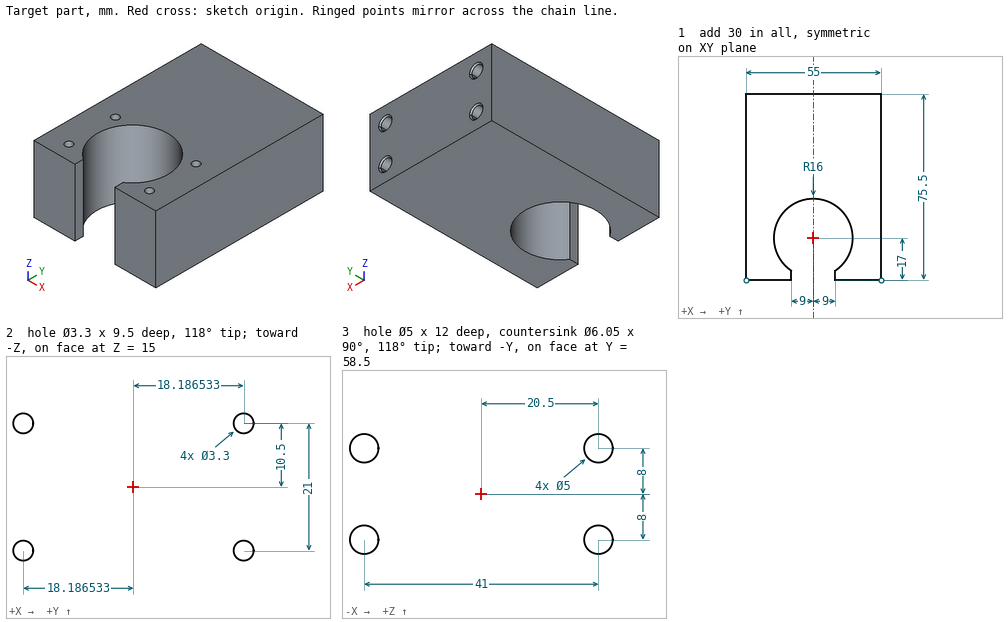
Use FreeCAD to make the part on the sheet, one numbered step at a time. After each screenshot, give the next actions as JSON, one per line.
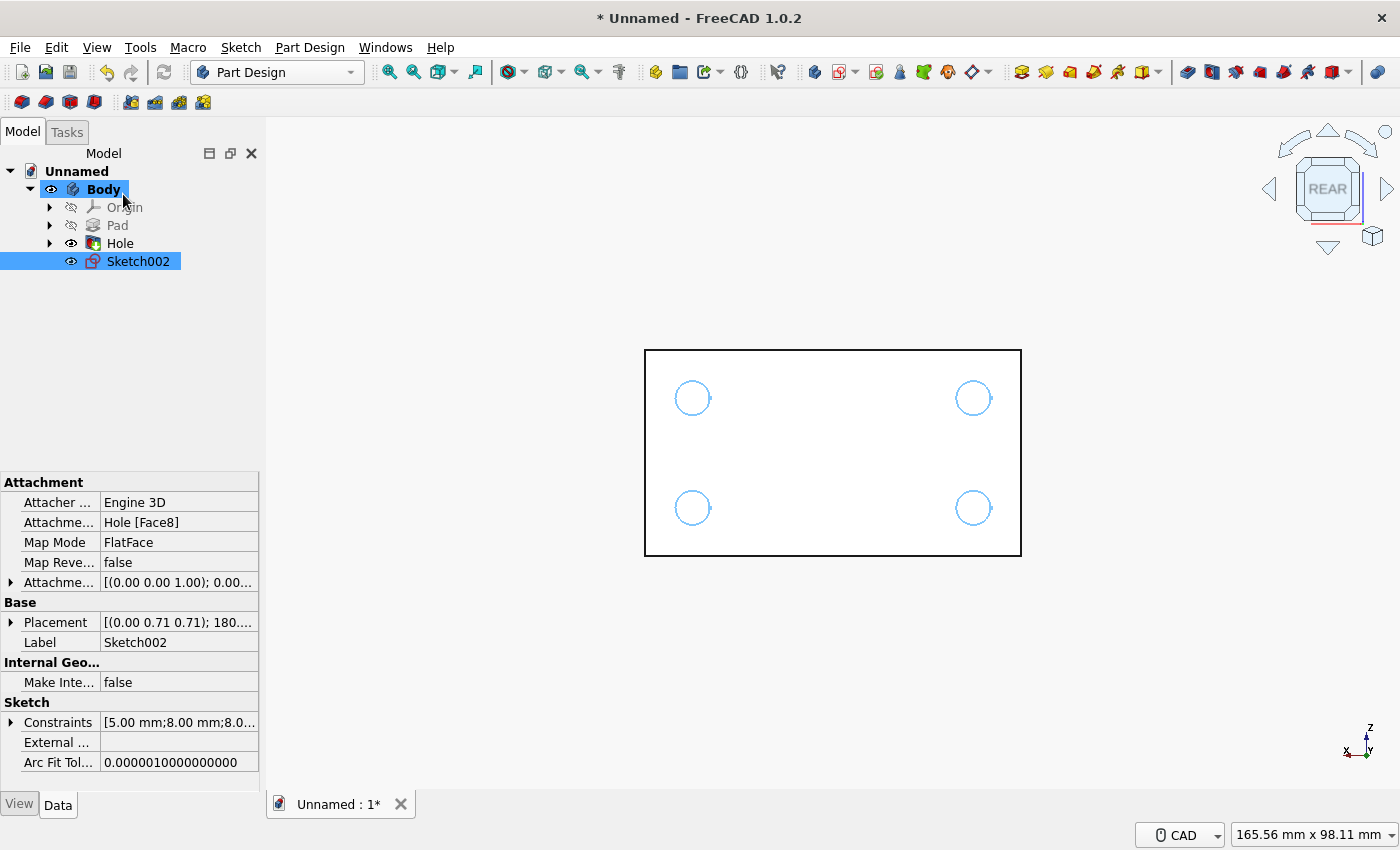
{"action": "left_click", "coordinate": [1212, 72]}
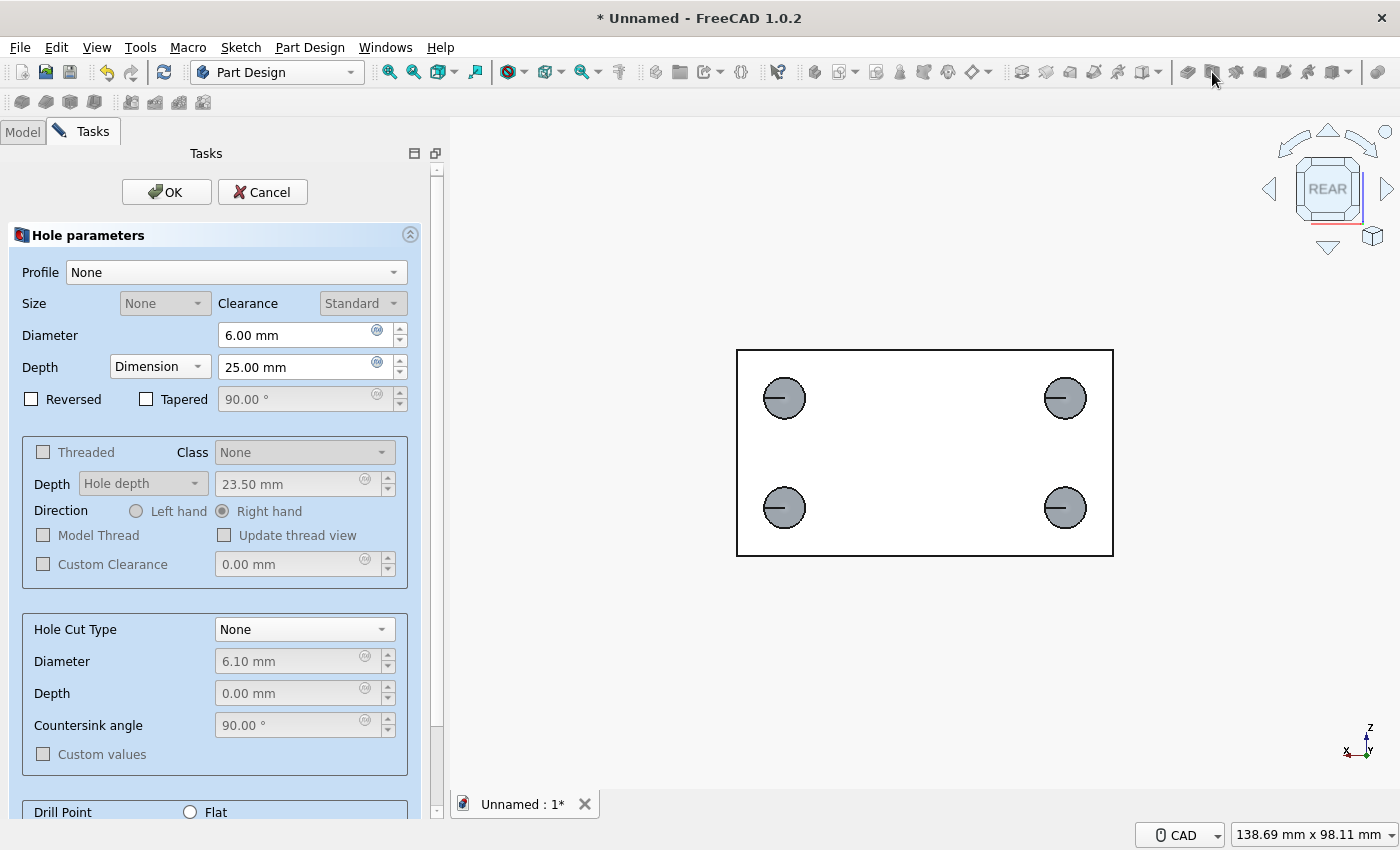
{"action": "triple_click", "coordinate": [305, 335]}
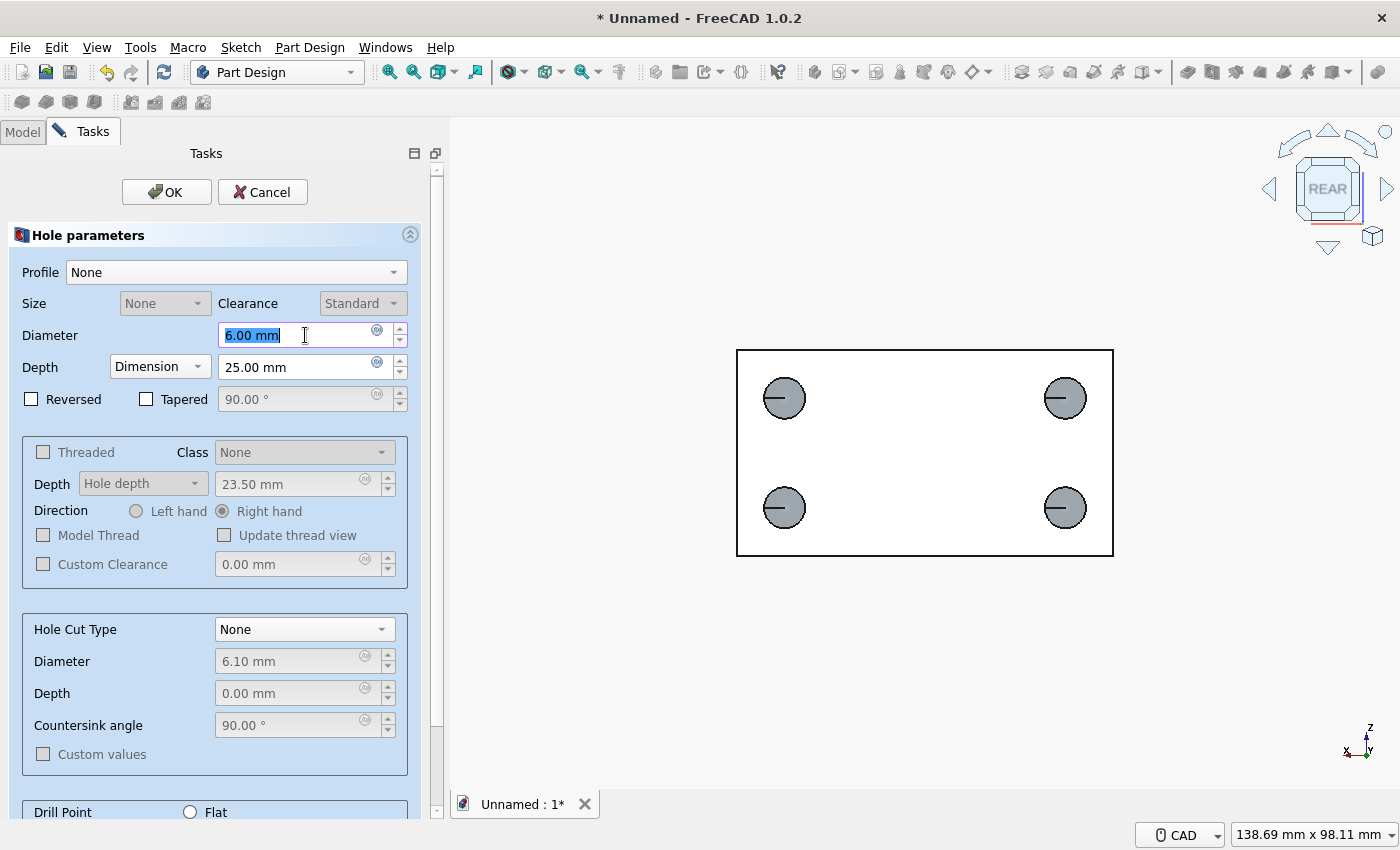
{"action": "type", "text": "5"}
{"action": "key", "text": "Tab"}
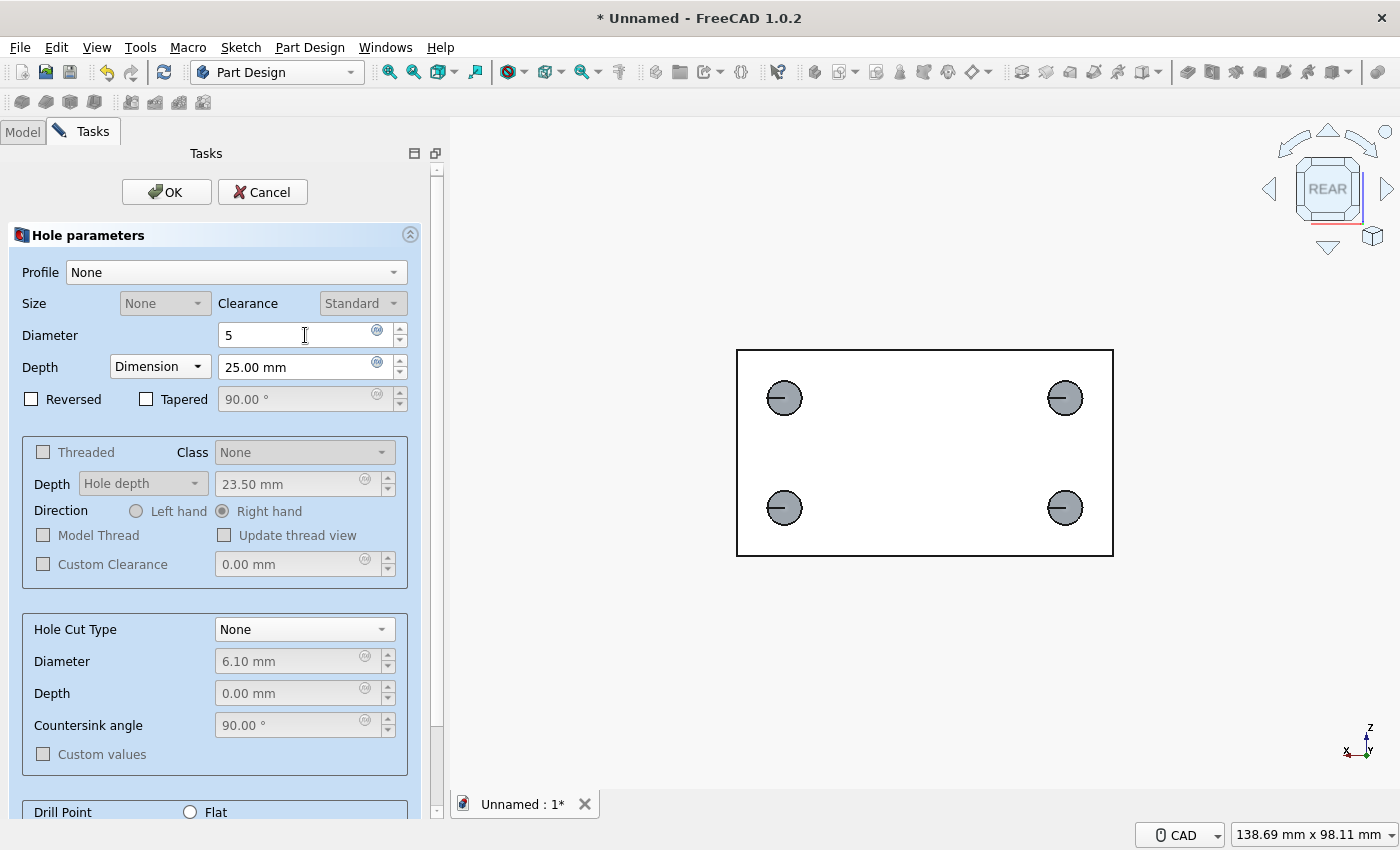
{"action": "triple_click", "coordinate": [305, 367]}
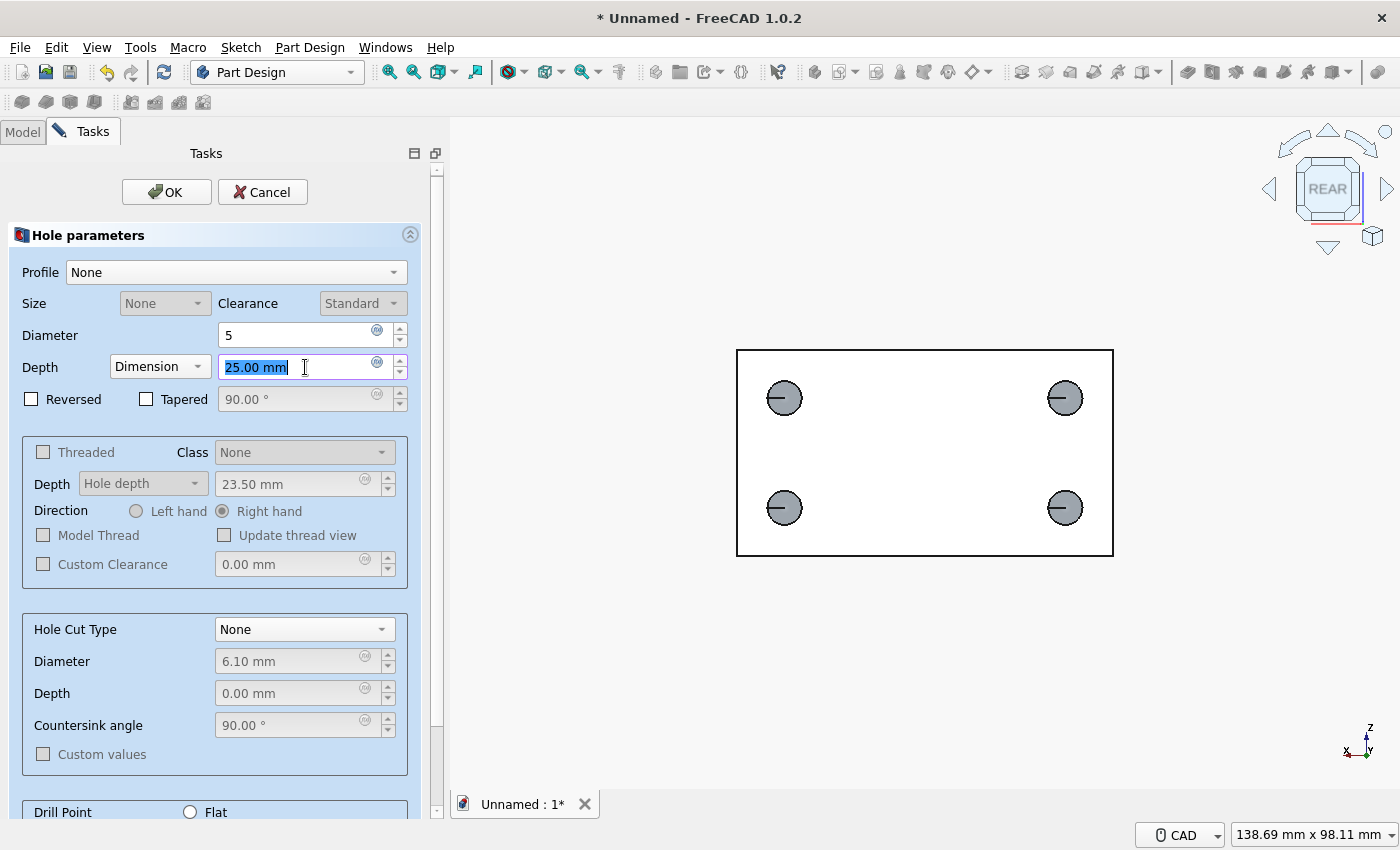
{"action": "type", "text": "12"}
{"action": "key", "text": "Tab"}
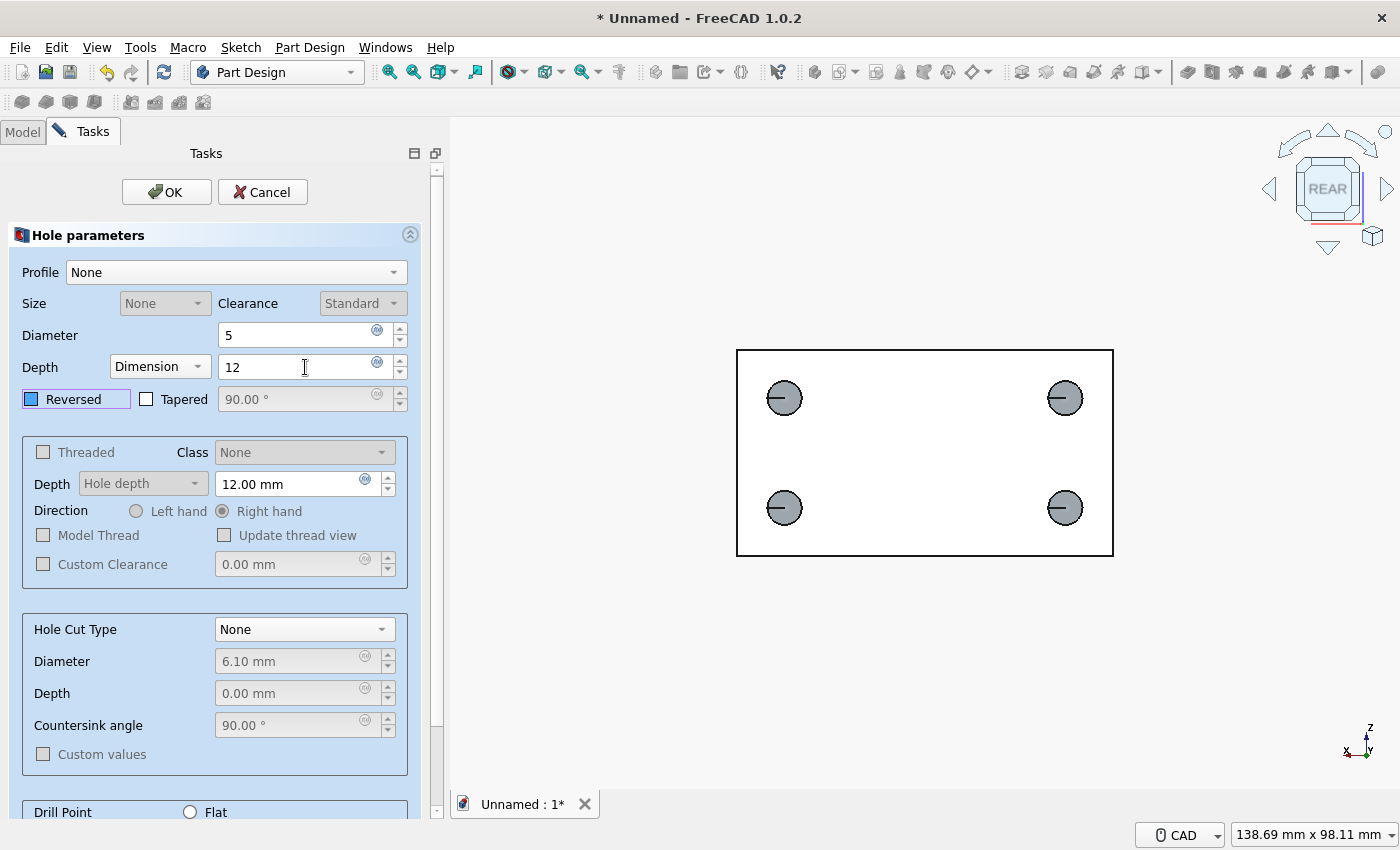
{"action": "left_click", "coordinate": [306, 630]}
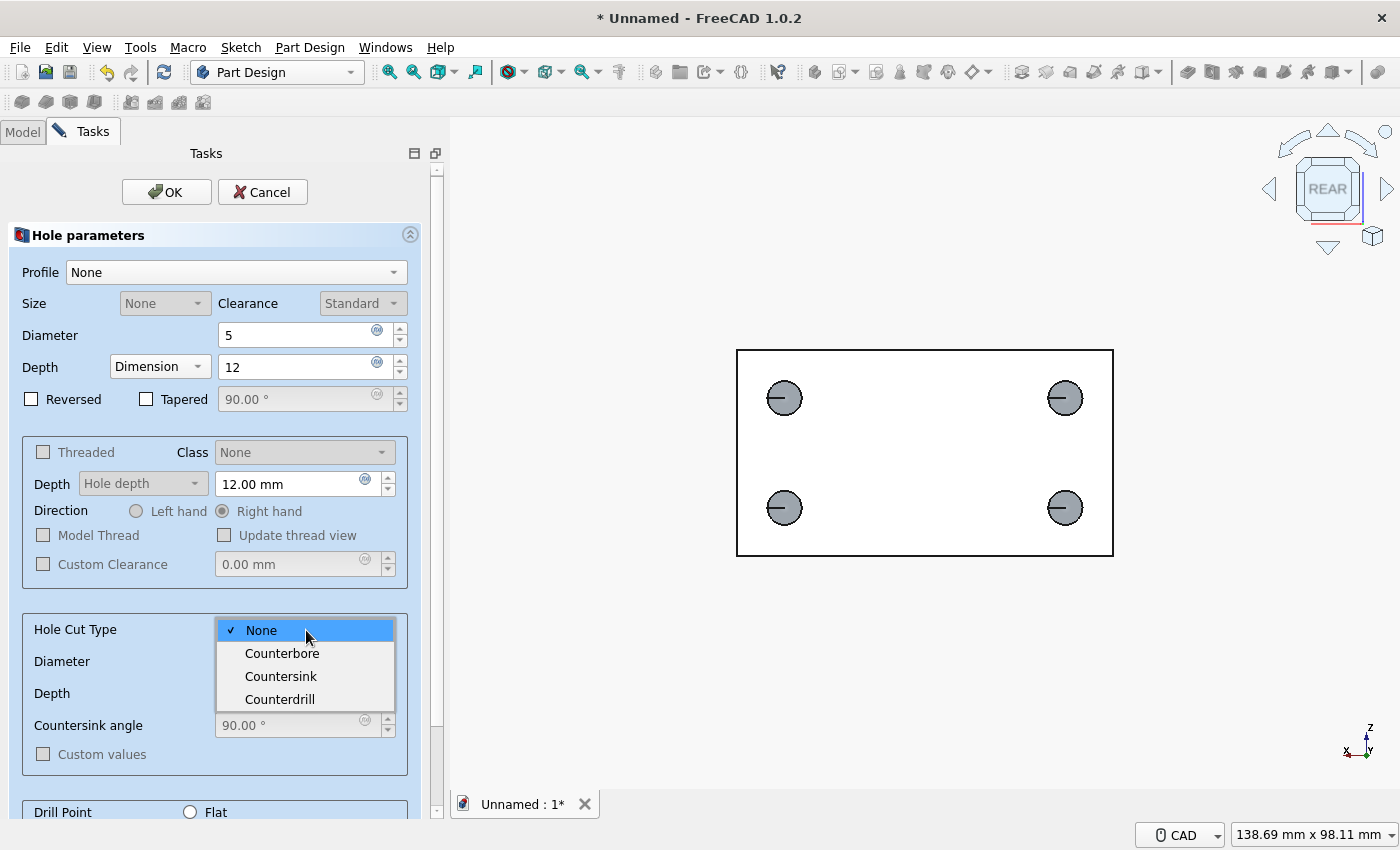
{"action": "left_click", "coordinate": [304, 676]}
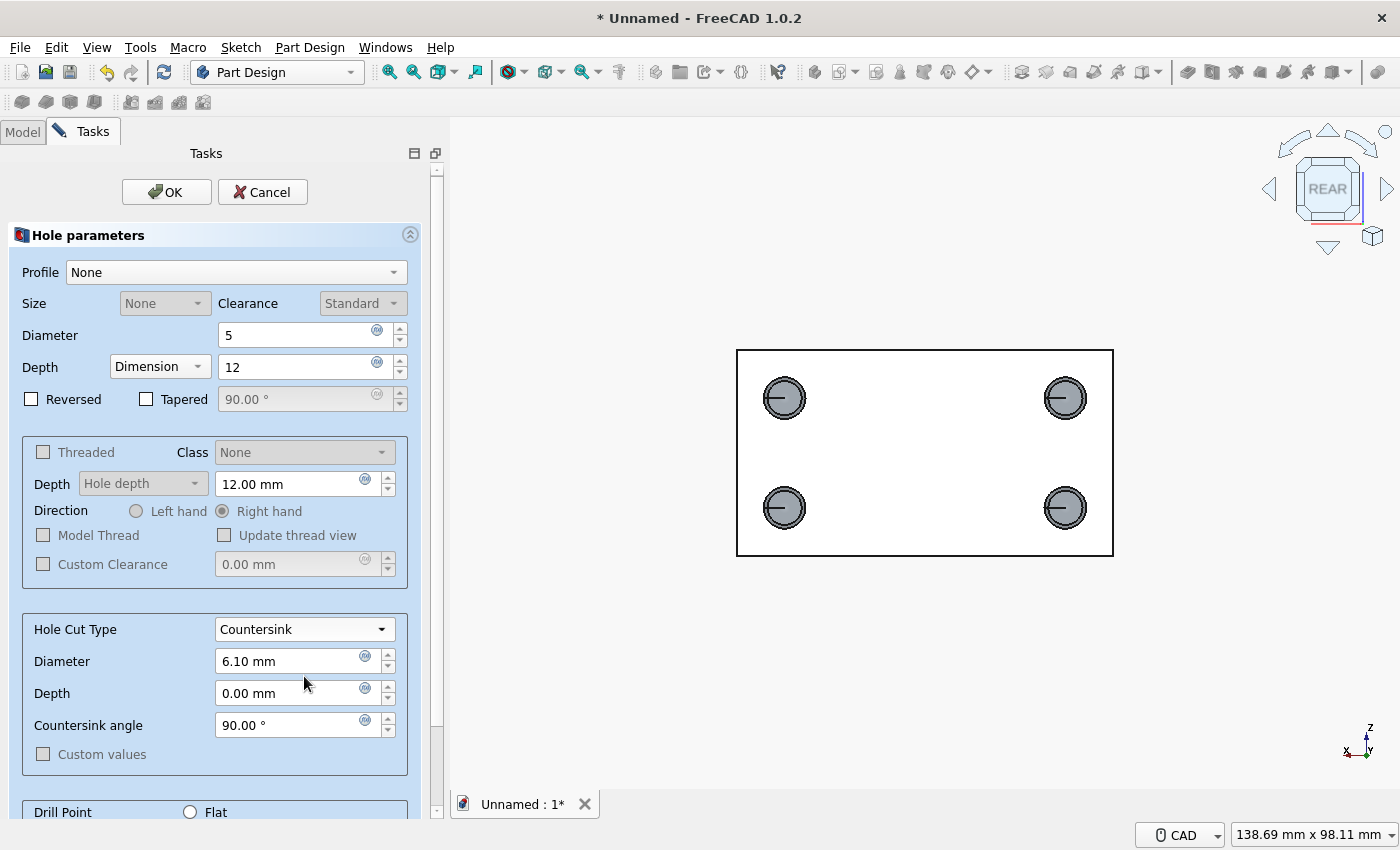
{"action": "triple_click", "coordinate": [298, 661]}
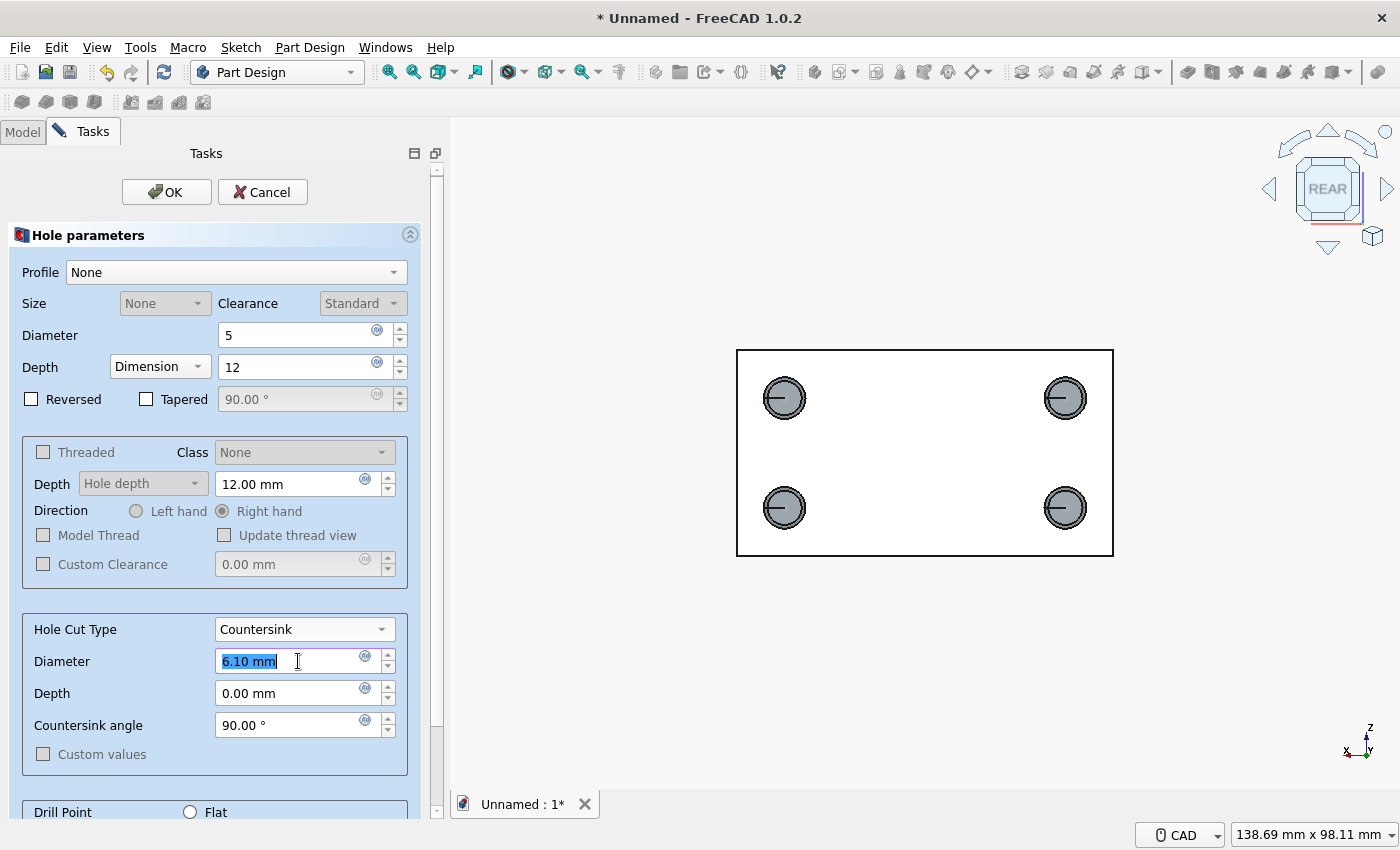
{"action": "type", "text": "6.05"}
{"action": "key", "text": "Tab"}